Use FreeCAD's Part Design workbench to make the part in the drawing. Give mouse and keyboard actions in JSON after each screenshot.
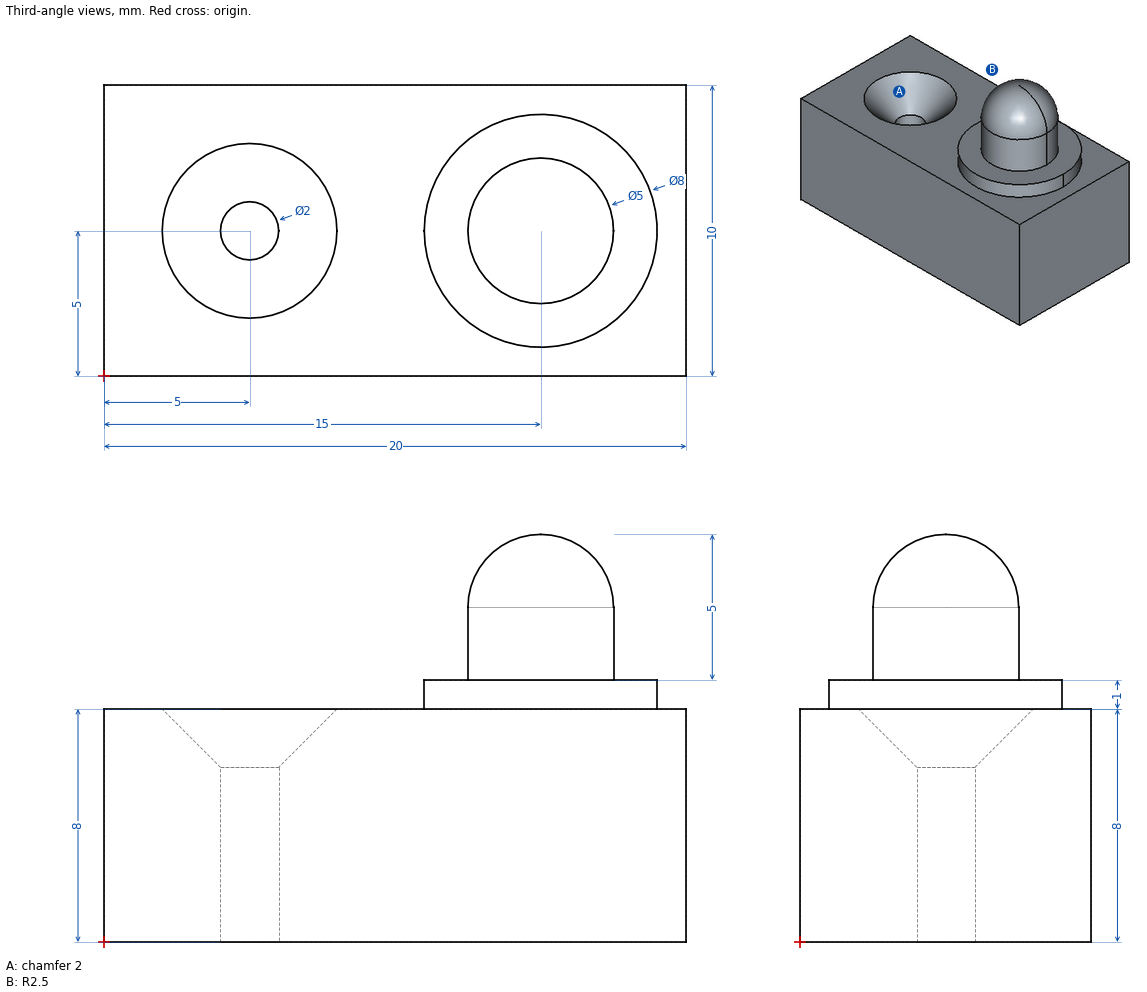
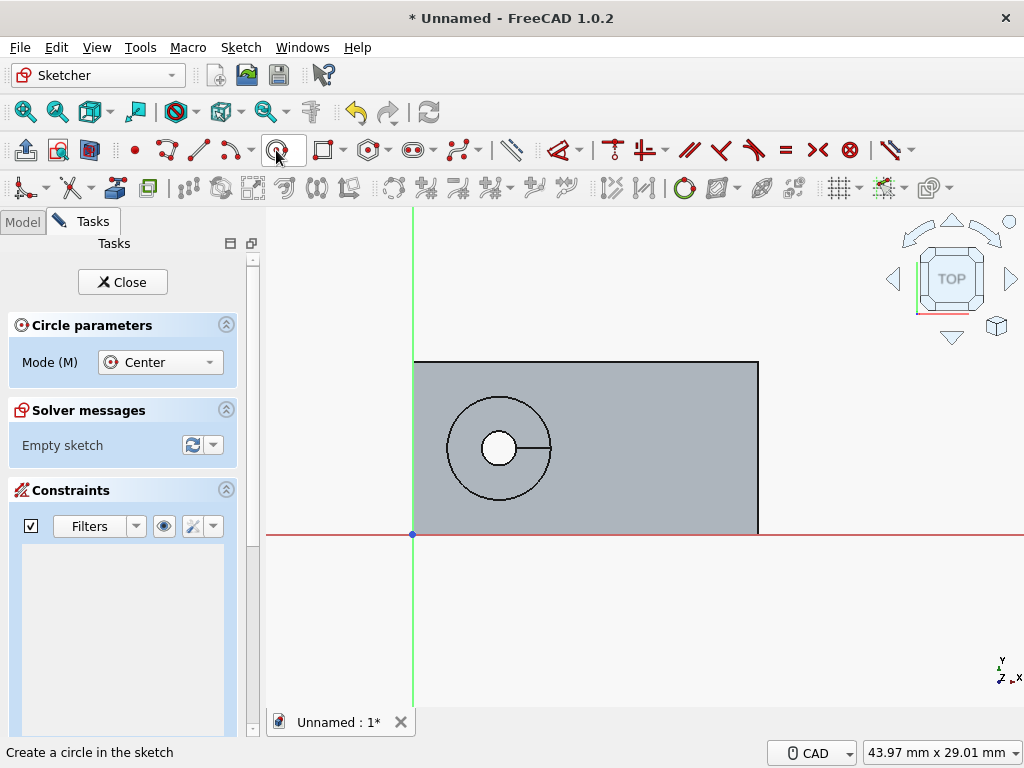
{"action": "left_click", "coordinate": [671, 448]}
{"action": "mouse_move", "coordinate": [720, 400]}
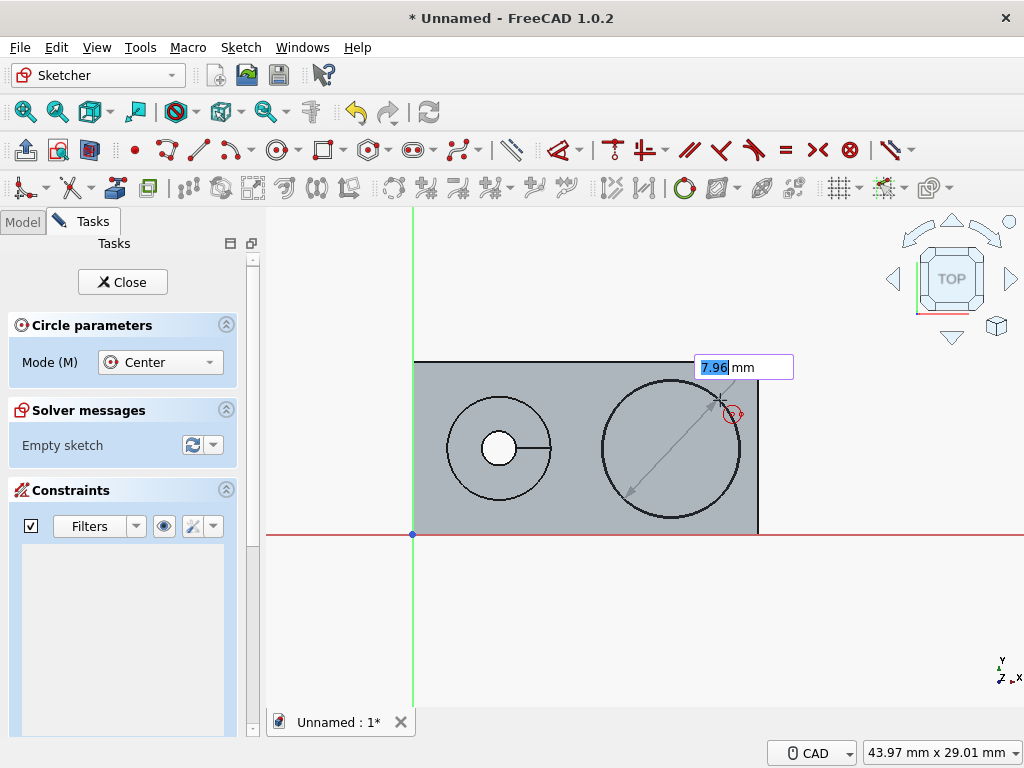
{"action": "type", "text": "8"}
{"action": "key", "text": "Return"}
{"action": "key", "text": "Escape"}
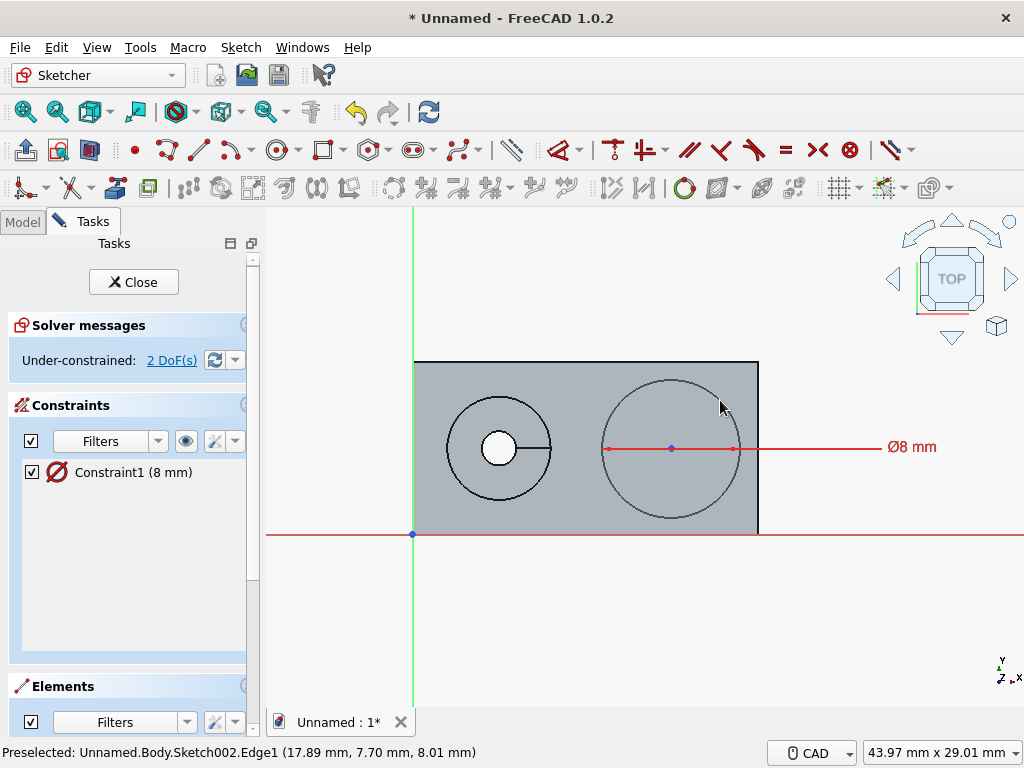
{"action": "left_click", "coordinate": [558, 150]}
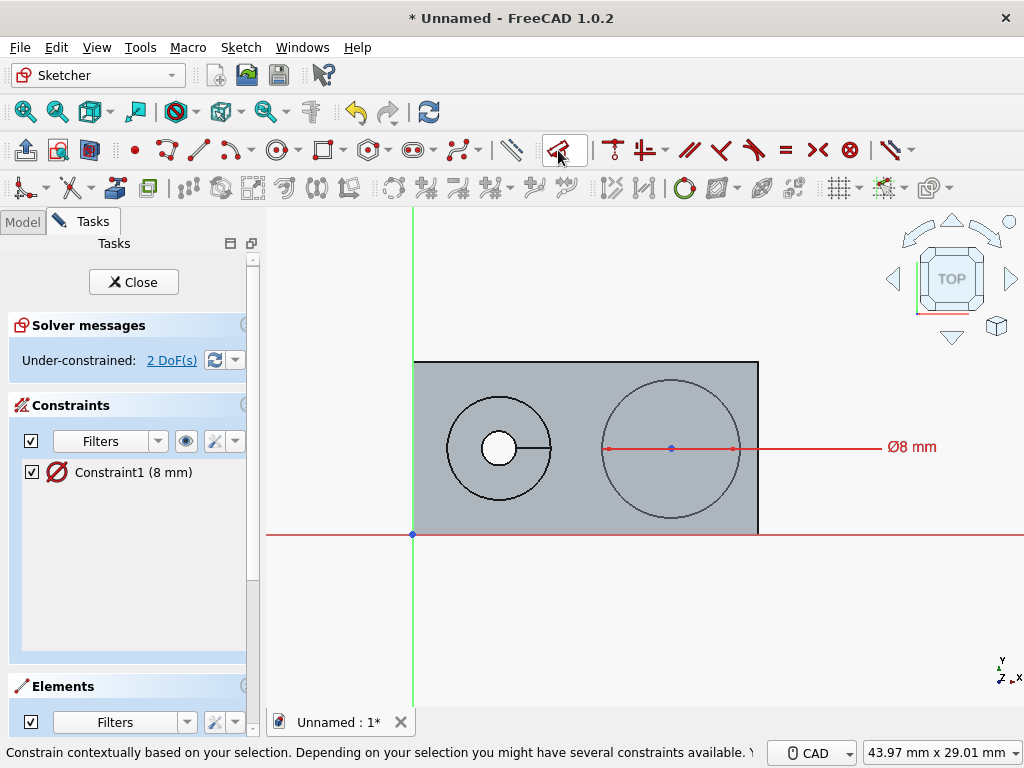
{"action": "left_click", "coordinate": [671, 449]}
{"action": "left_click", "coordinate": [379, 492]}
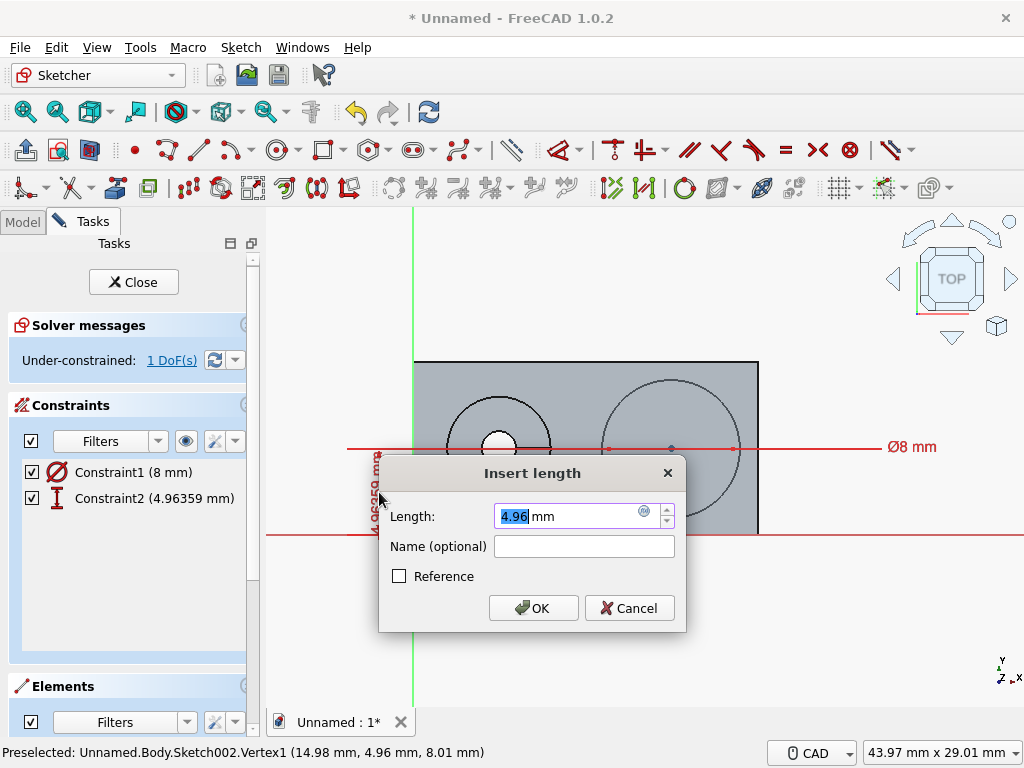
{"action": "type", "text": "5"}
{"action": "key", "text": "Return"}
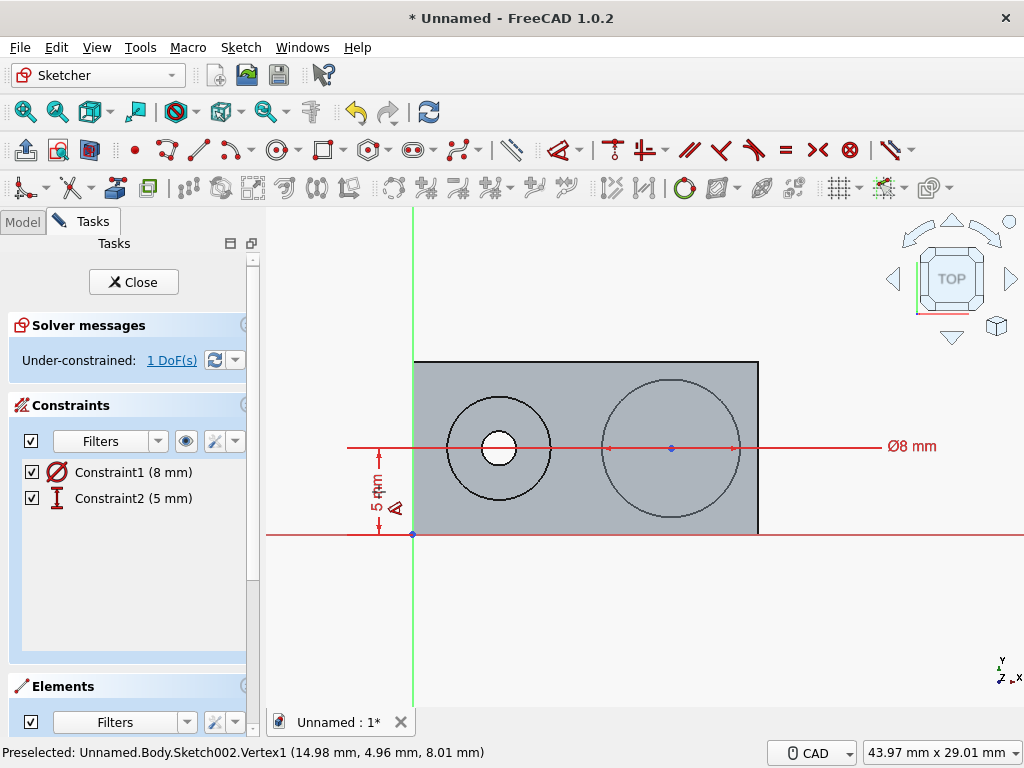
{"action": "left_click", "coordinate": [671, 448]}
{"action": "left_click", "coordinate": [542, 569]}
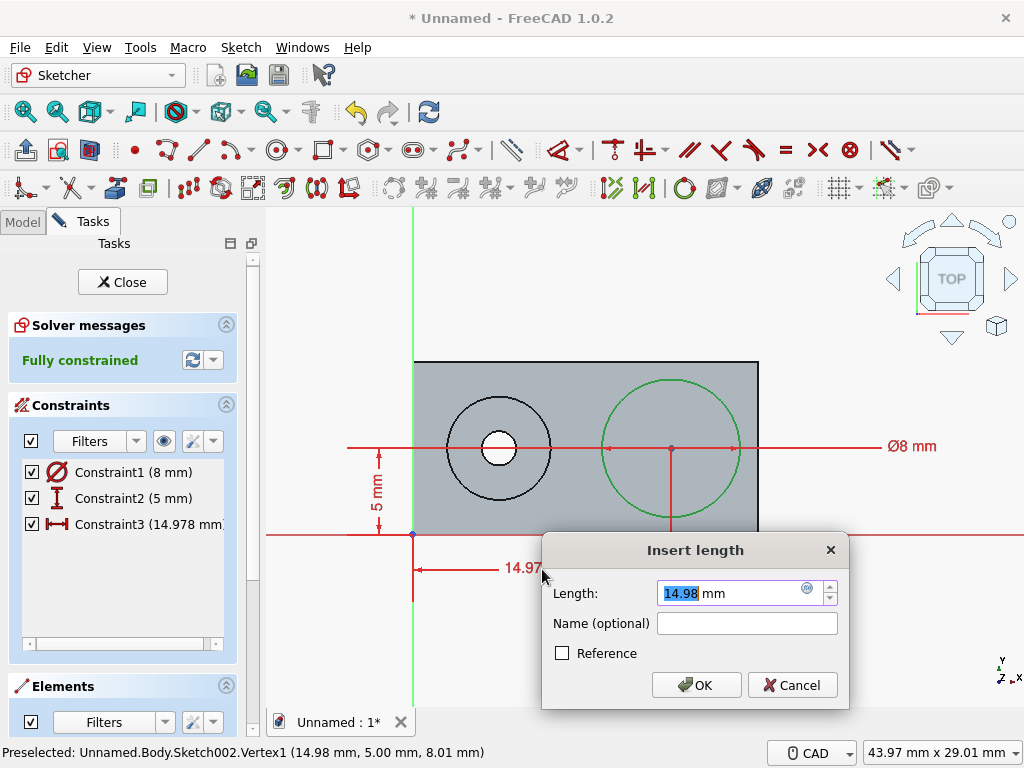
{"action": "type", "text": "15"}
{"action": "key", "text": "Return"}
{"action": "key", "text": "Escape"}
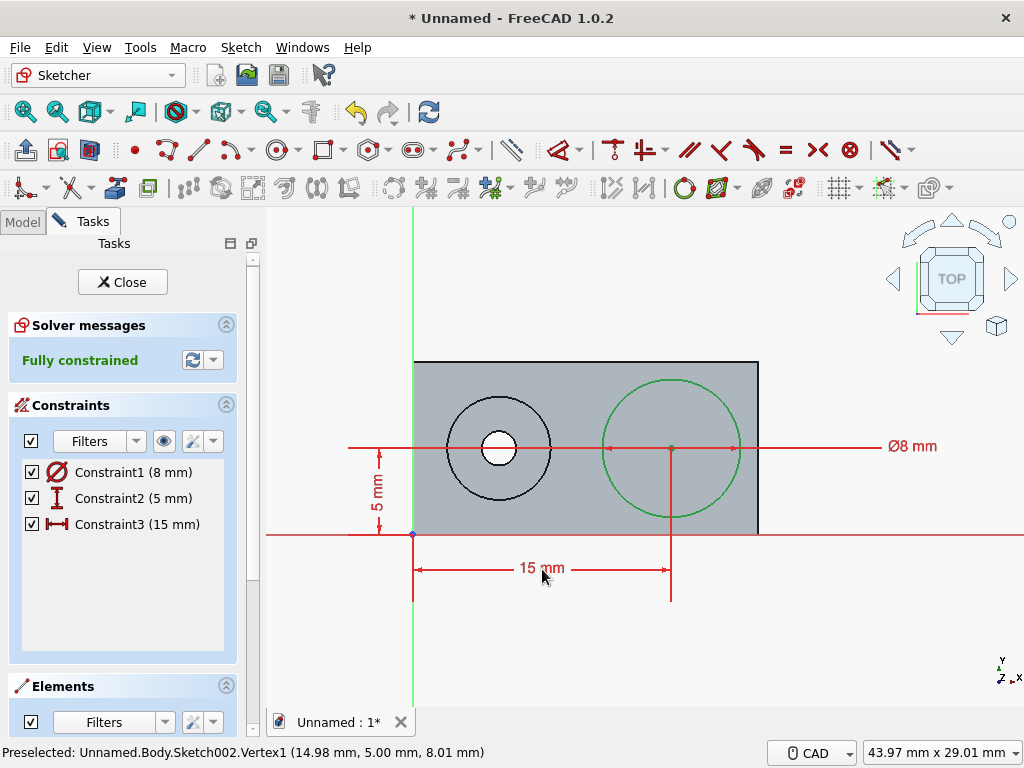
{"action": "left_click", "coordinate": [123, 282]}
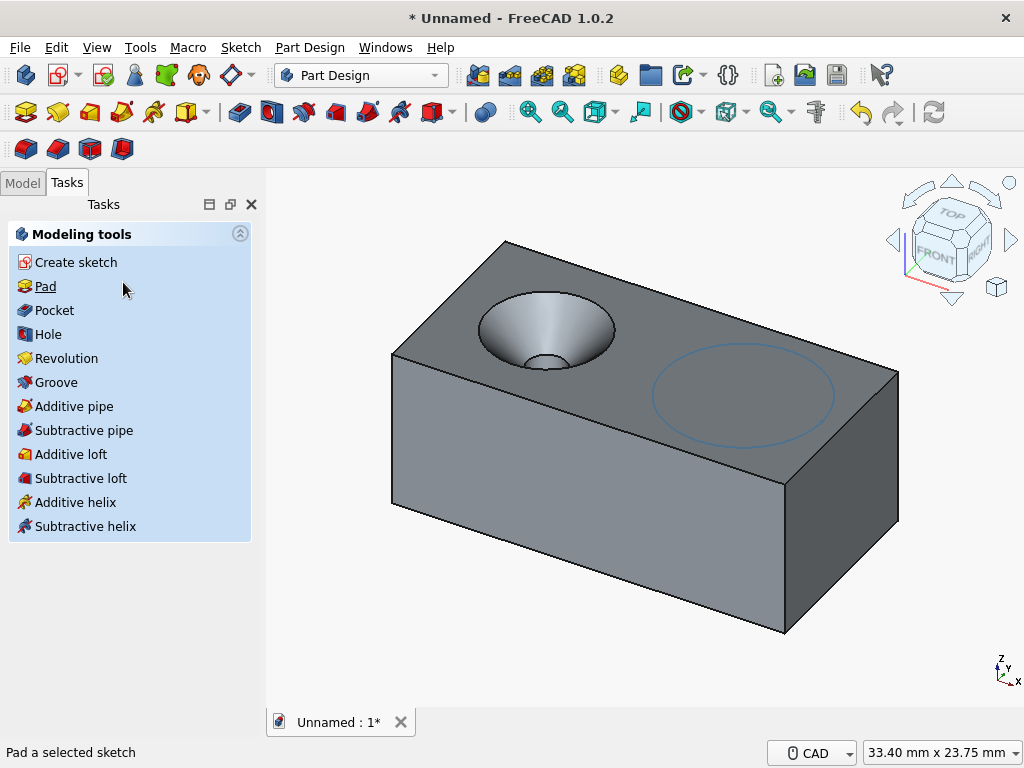
{"action": "left_click", "coordinate": [26, 112]}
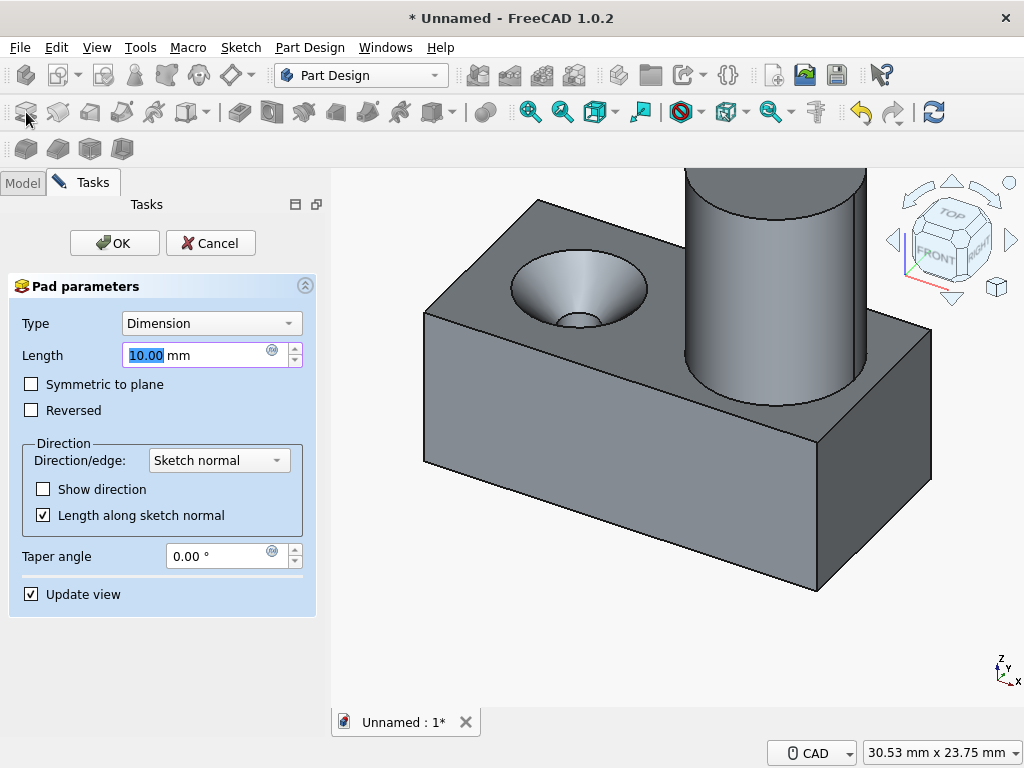
{"action": "type", "text": "1"}
{"action": "key", "text": "Tab"}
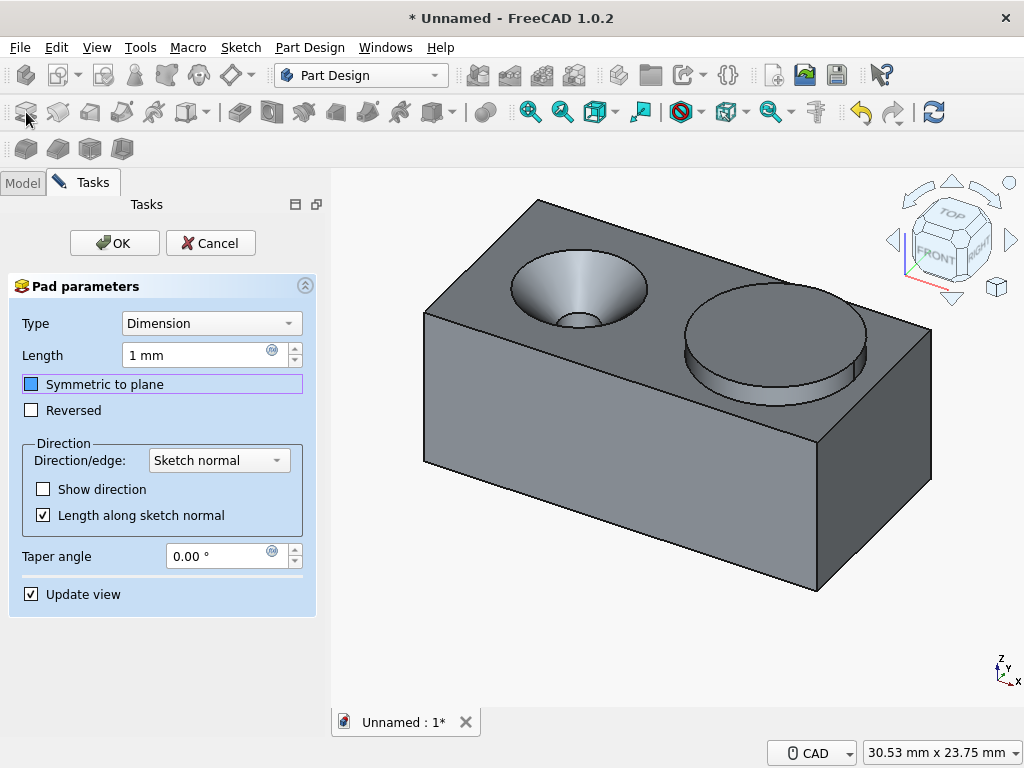
{"action": "left_click", "coordinate": [115, 243]}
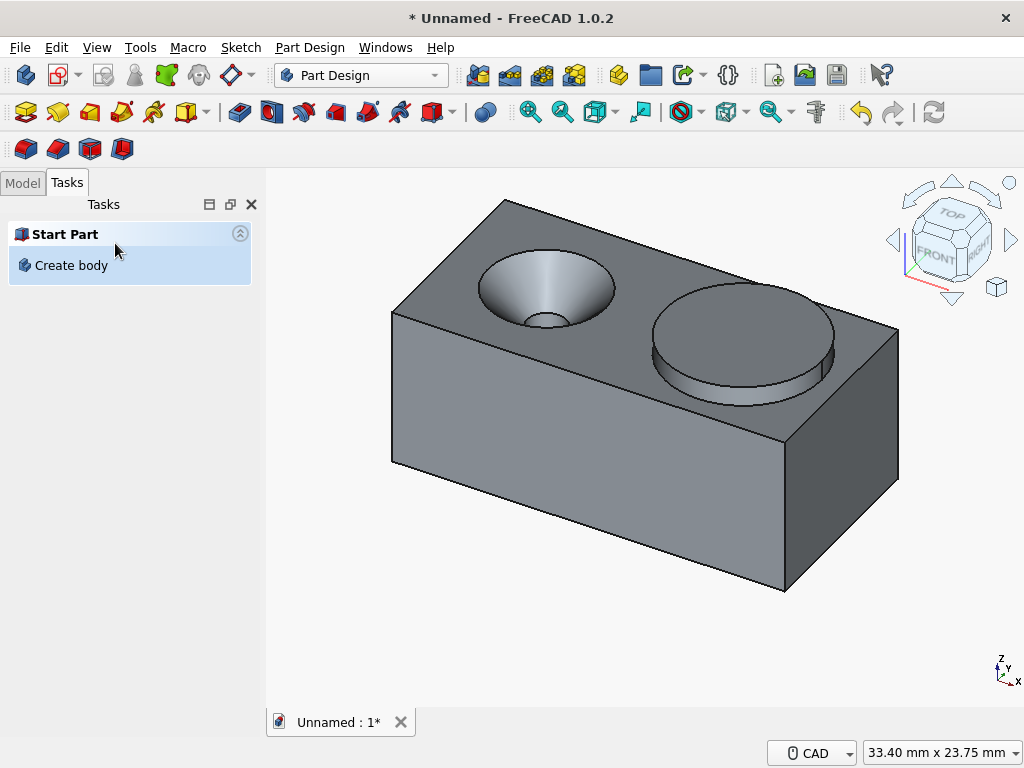
{"action": "left_click", "coordinate": [743, 334]}